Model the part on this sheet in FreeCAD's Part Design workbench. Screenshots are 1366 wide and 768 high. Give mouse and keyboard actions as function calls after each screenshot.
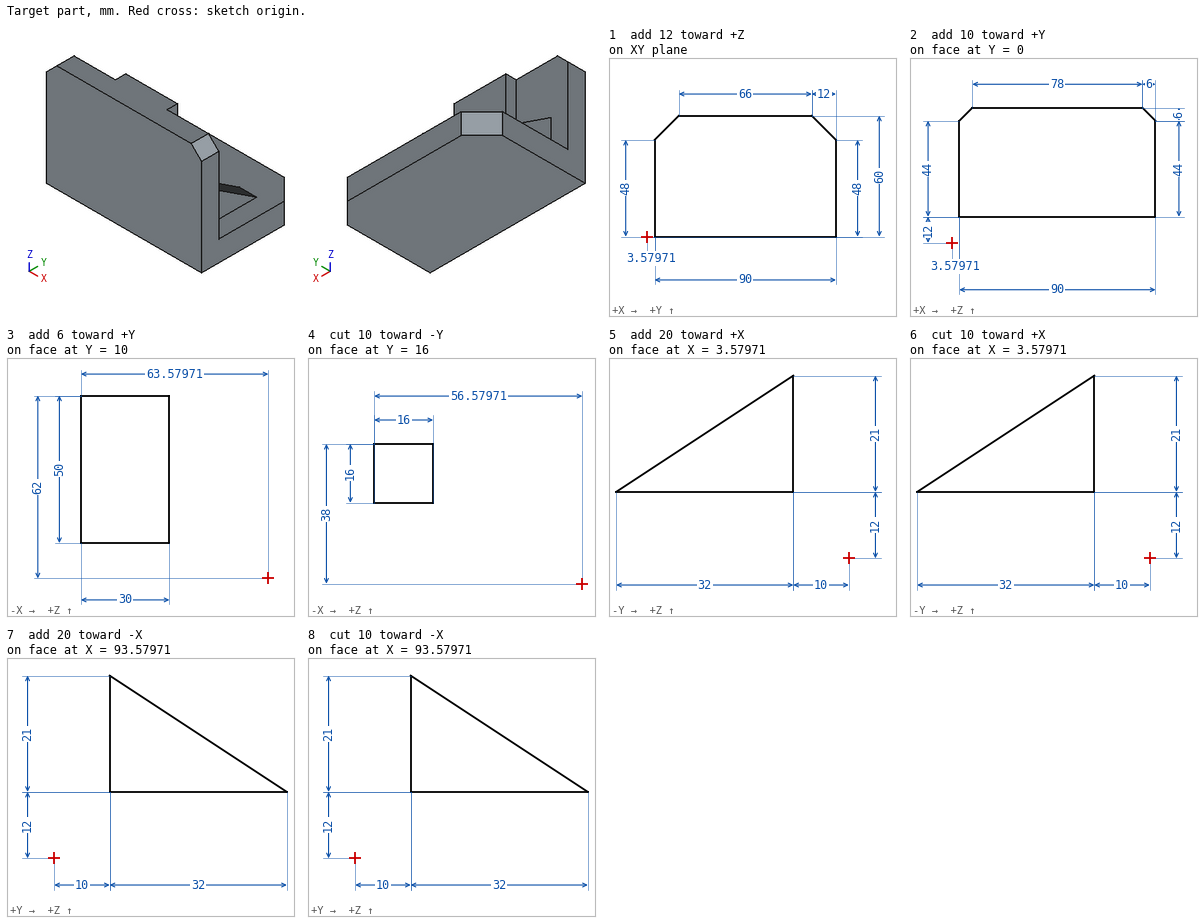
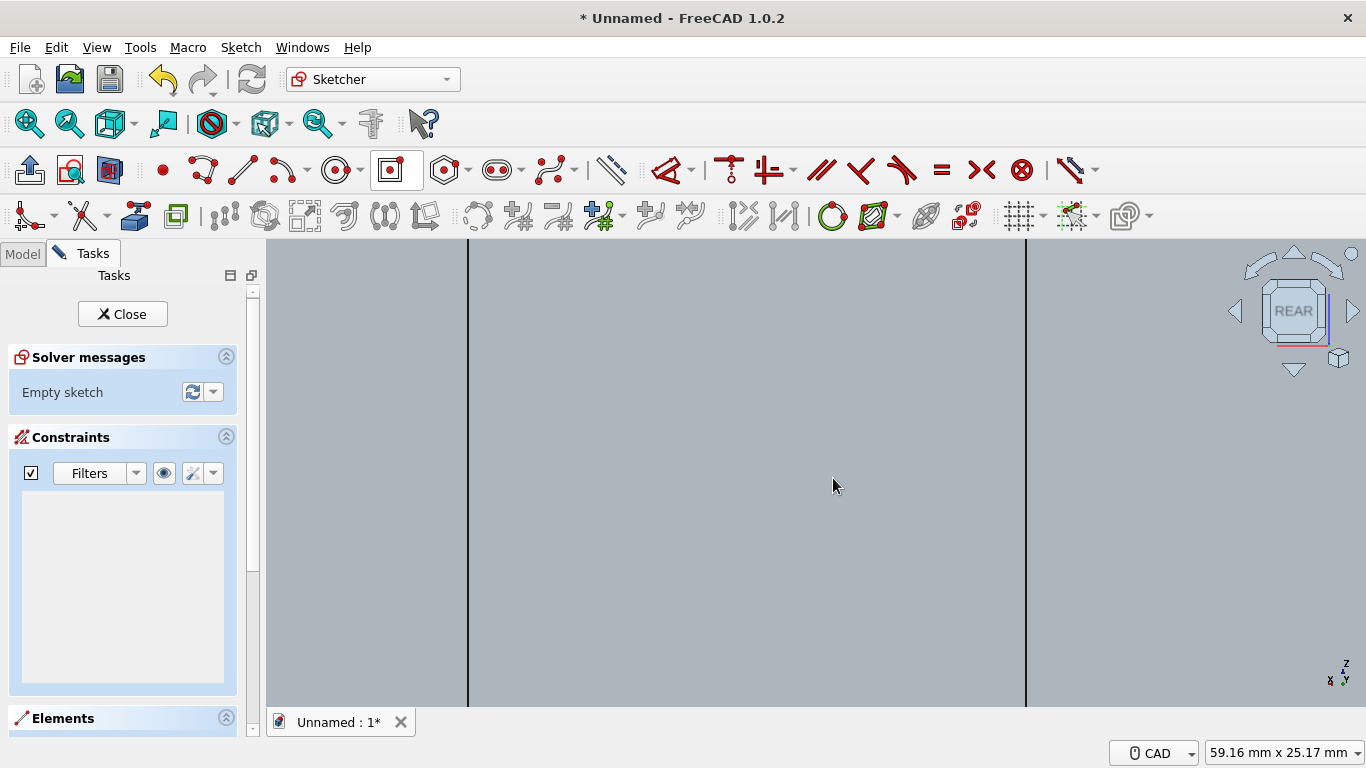
key(g)
key(r)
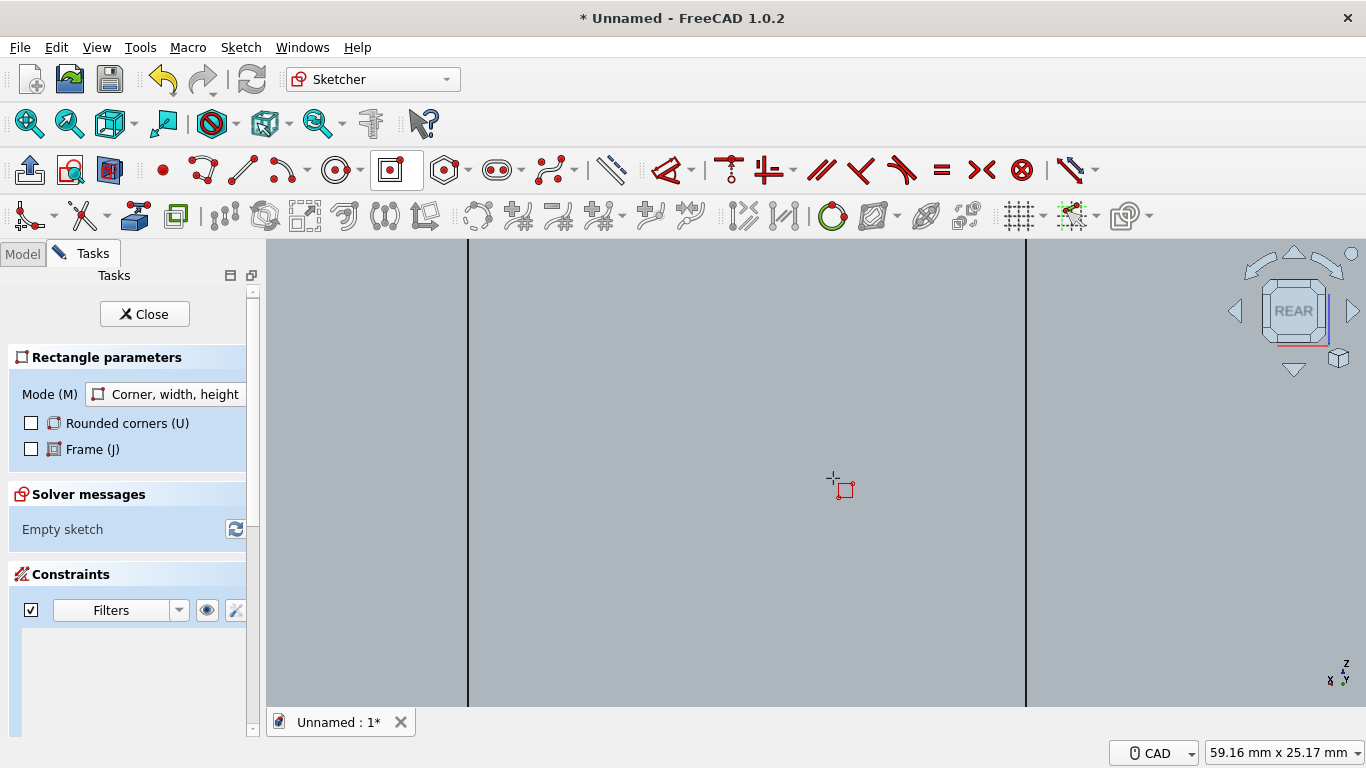
click(598, 321)
click(895, 619)
key(Escape)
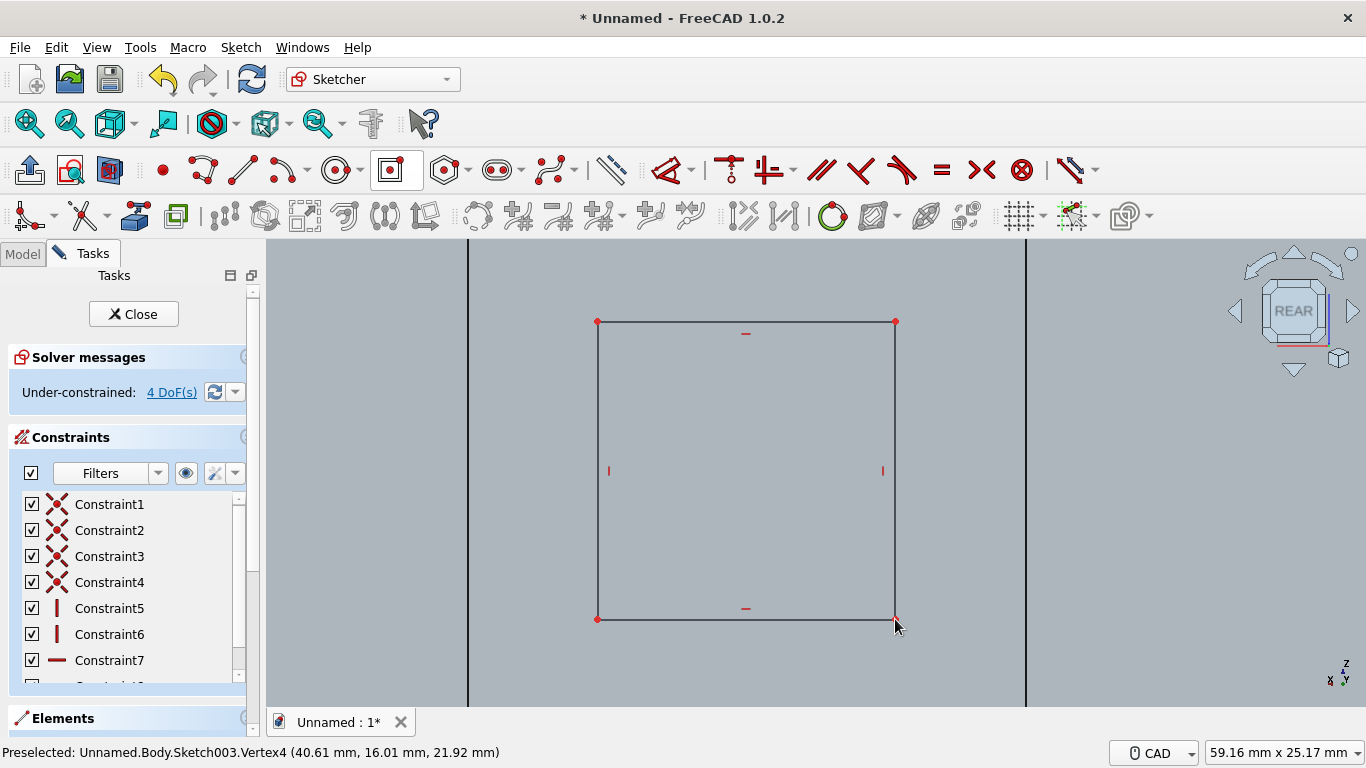
click(666, 170)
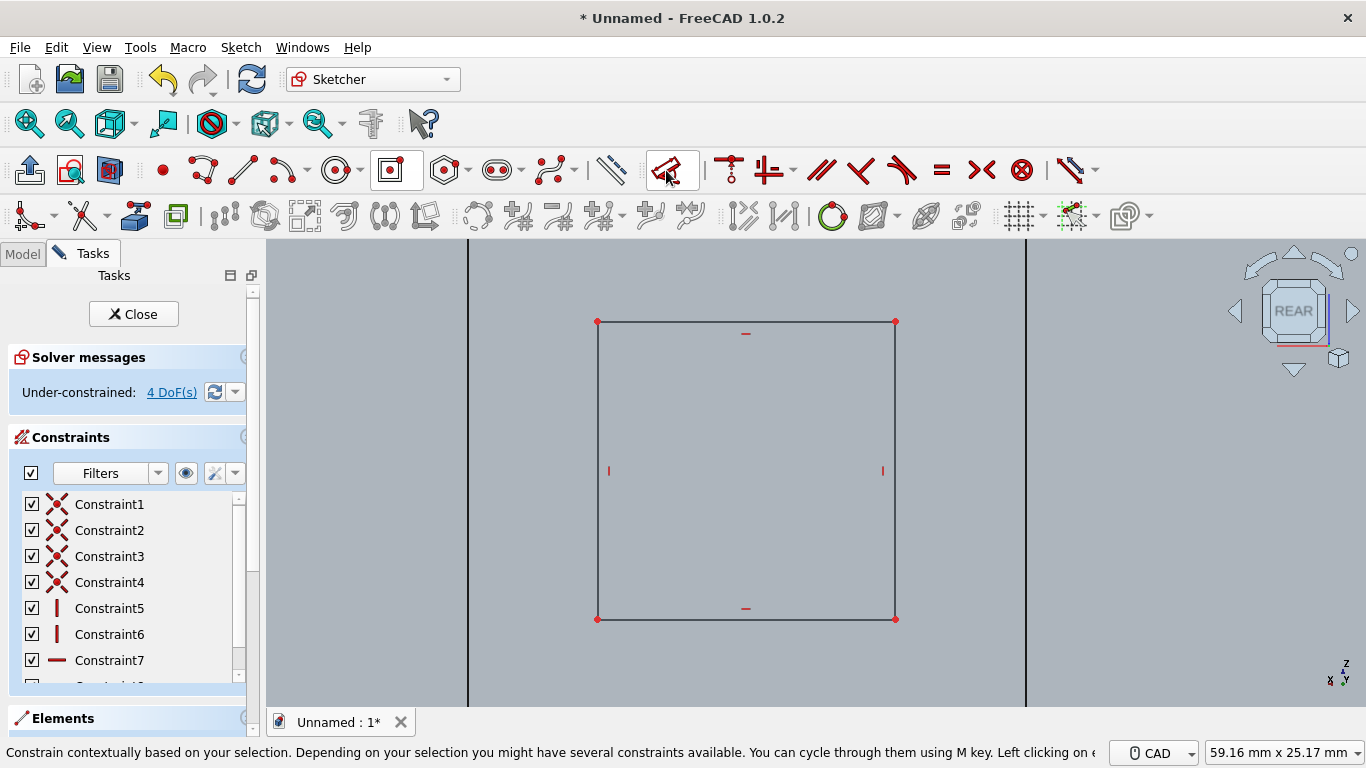
click(598, 411)
click(564, 471)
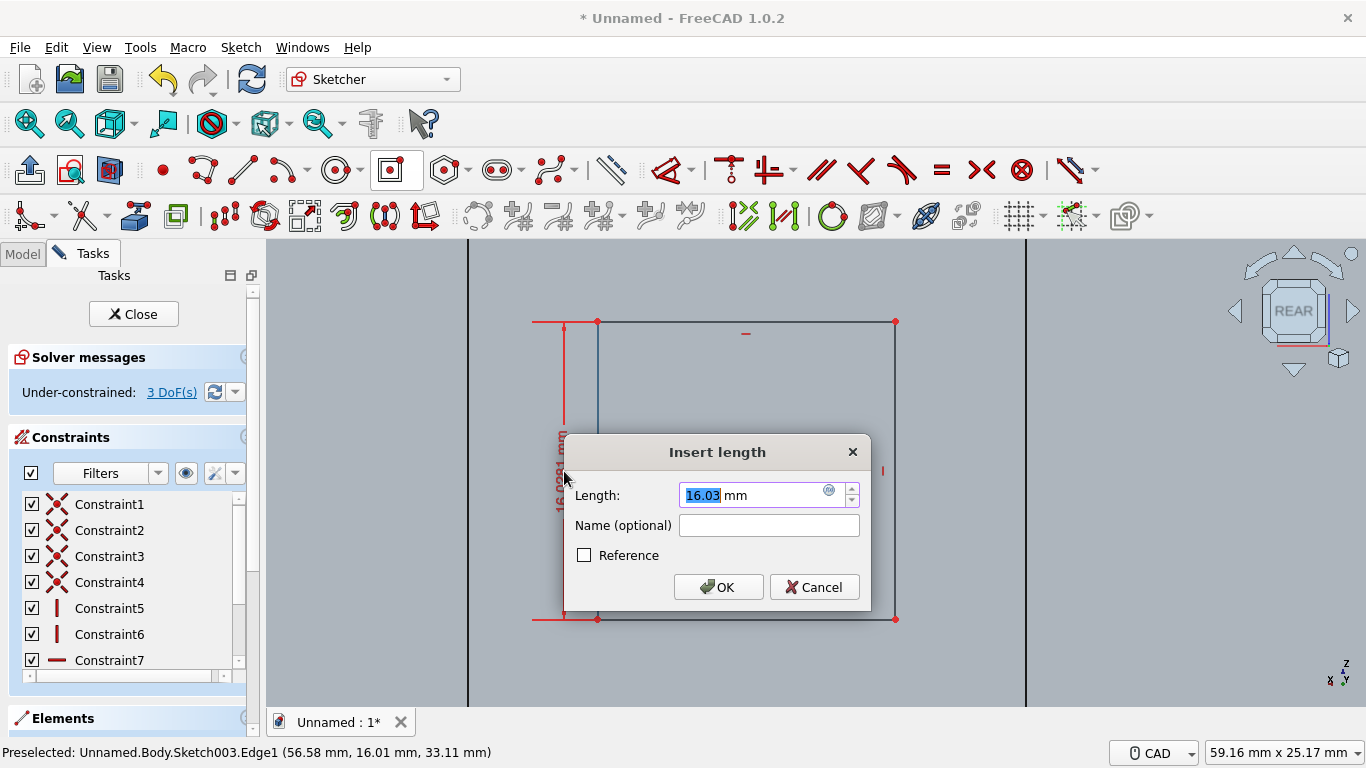
text(16)
key(Return)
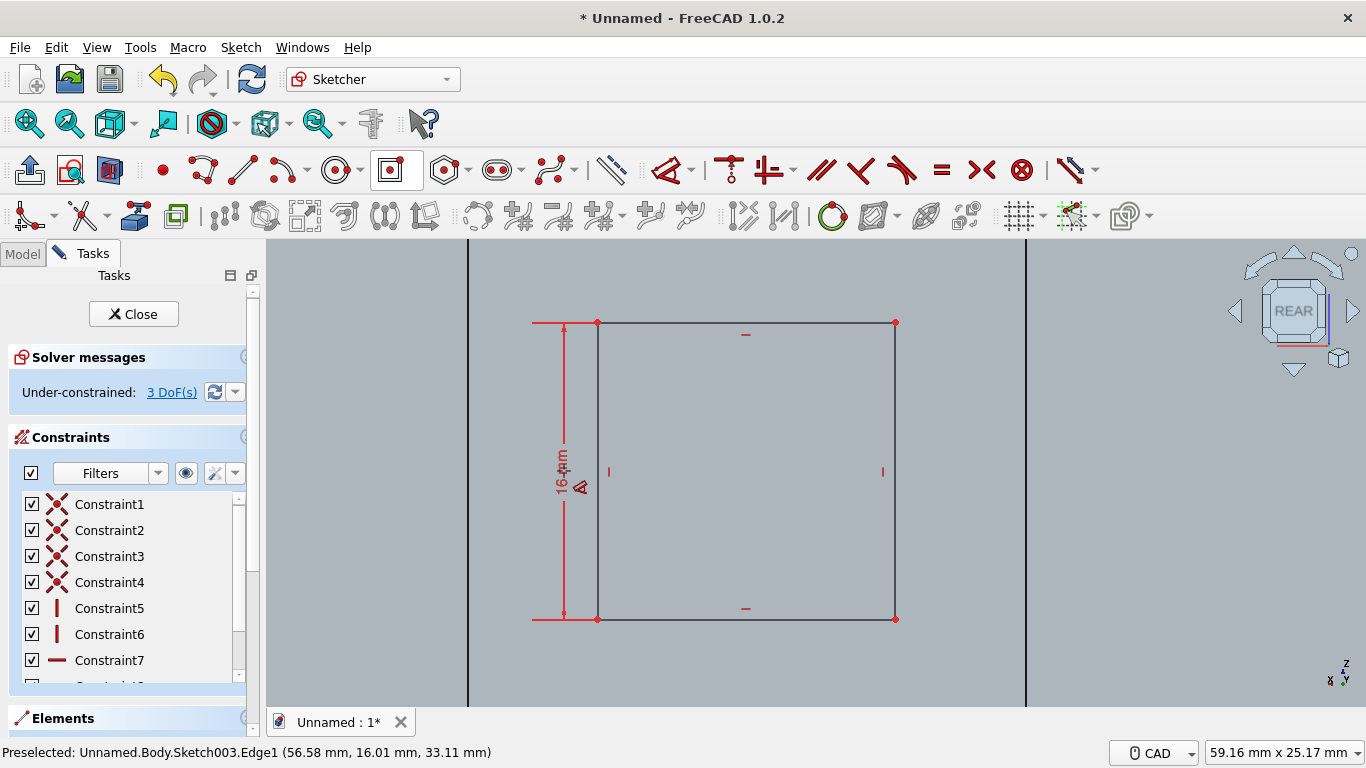
click(687, 620)
click(746, 654)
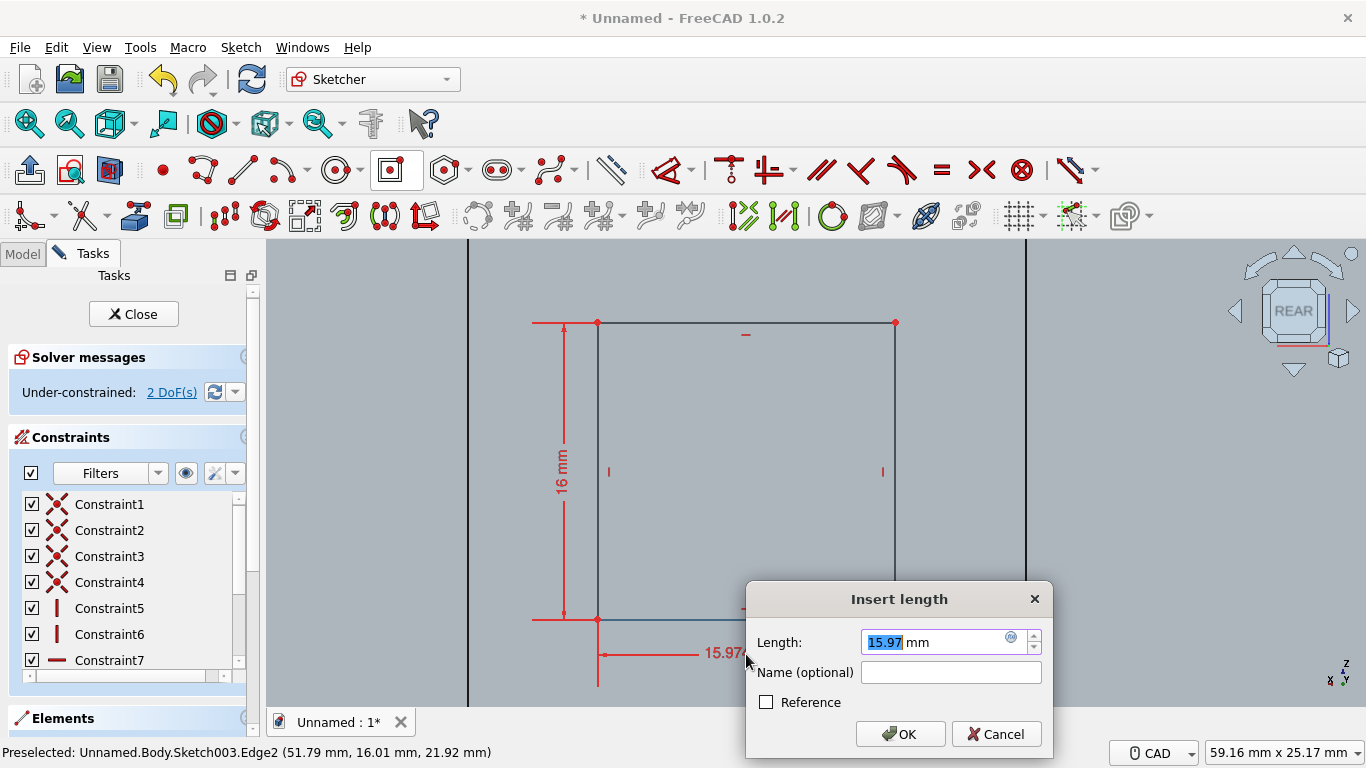
text(16)
key(Return)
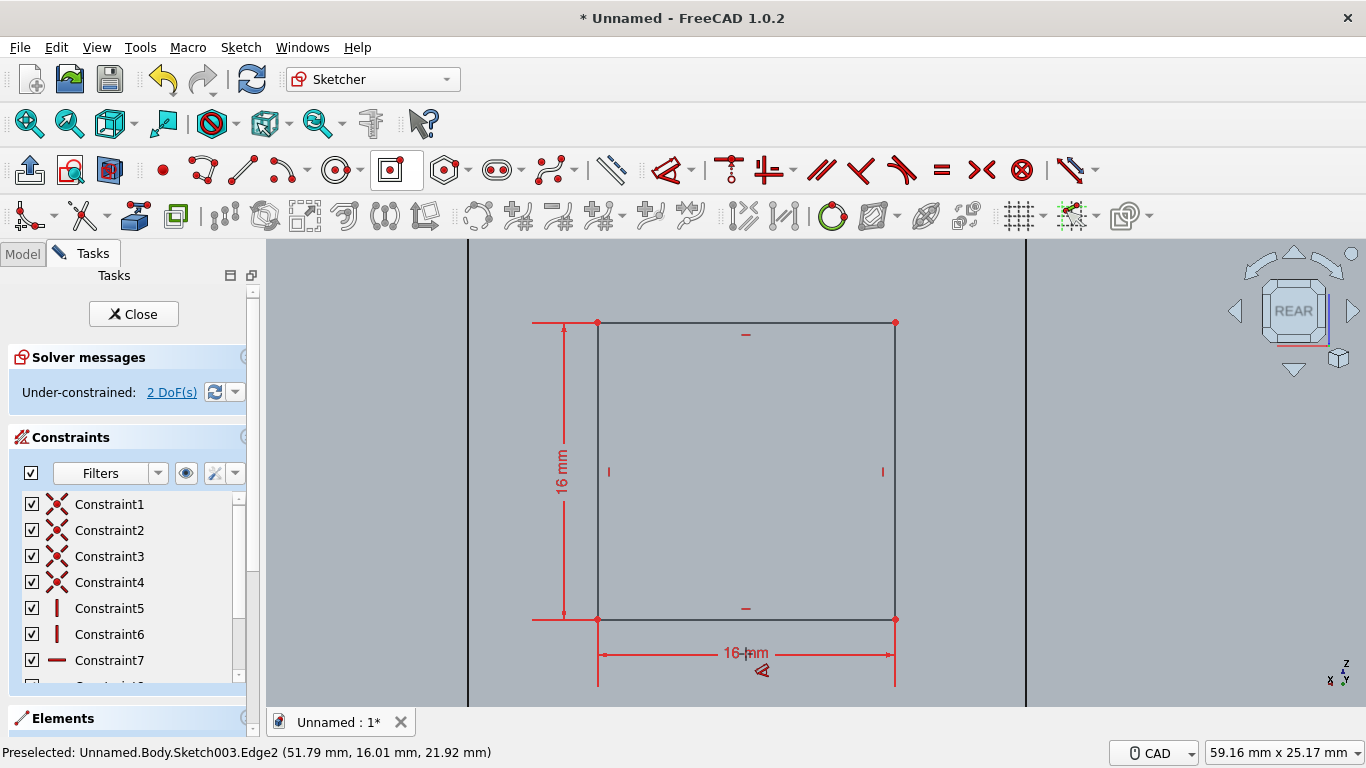
click(598, 323)
click(564, 501)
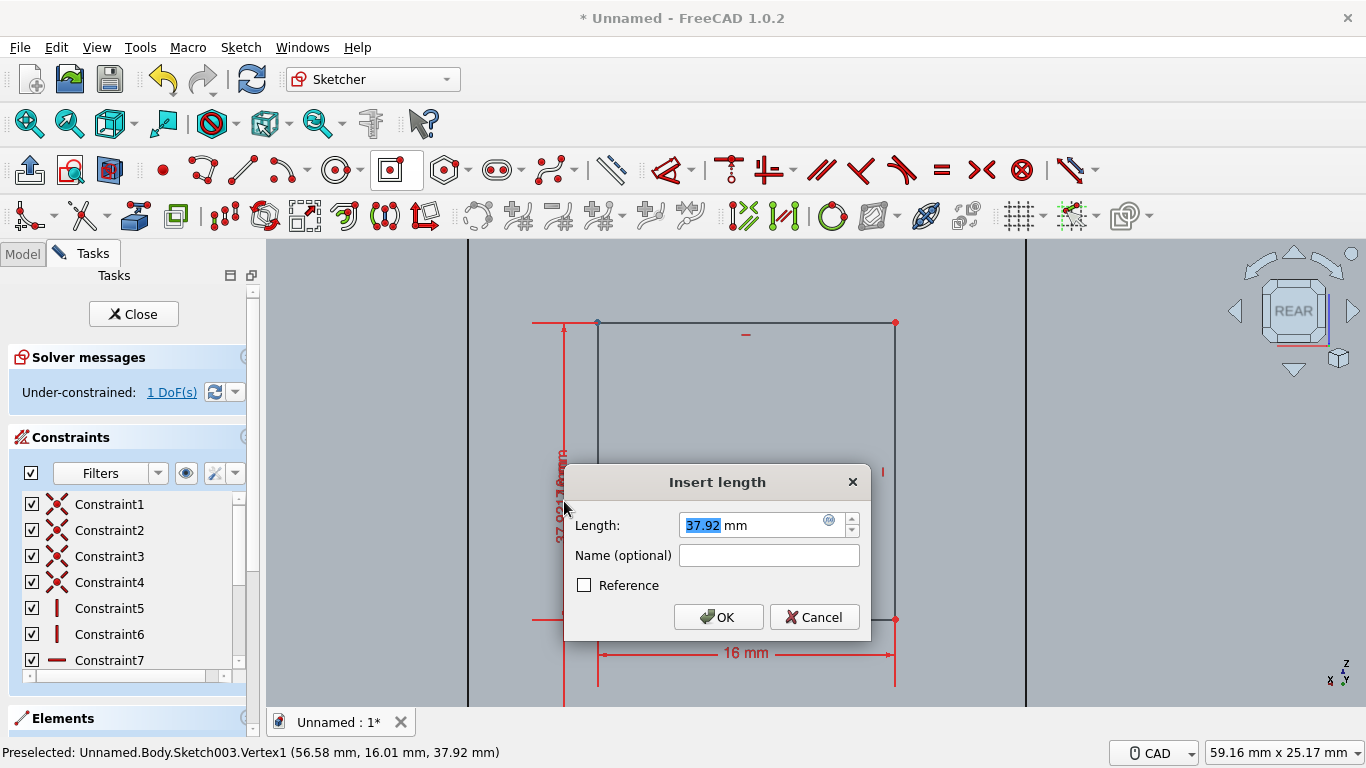
text(38)
key(Return)